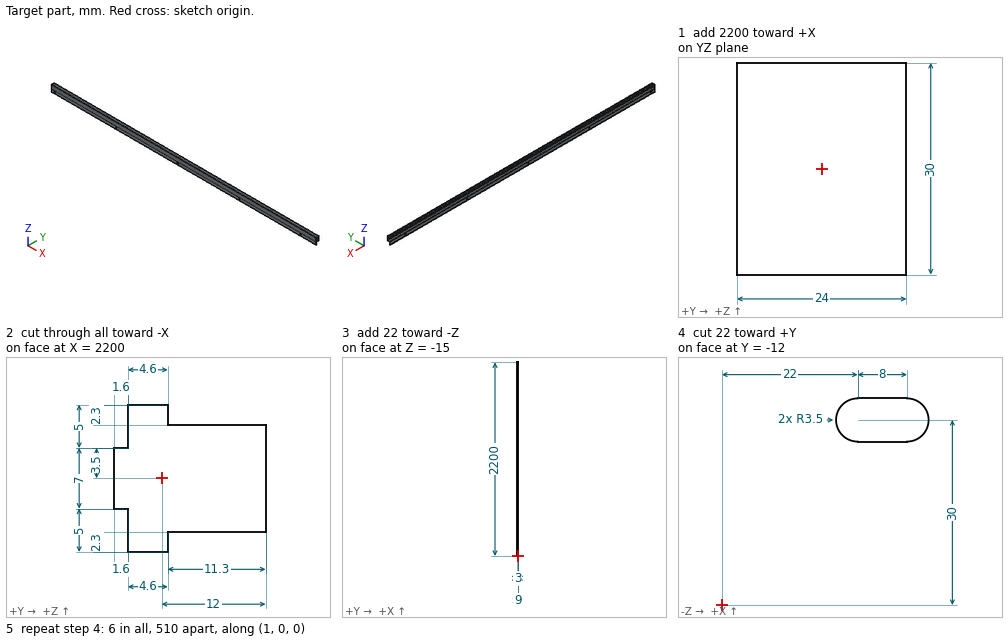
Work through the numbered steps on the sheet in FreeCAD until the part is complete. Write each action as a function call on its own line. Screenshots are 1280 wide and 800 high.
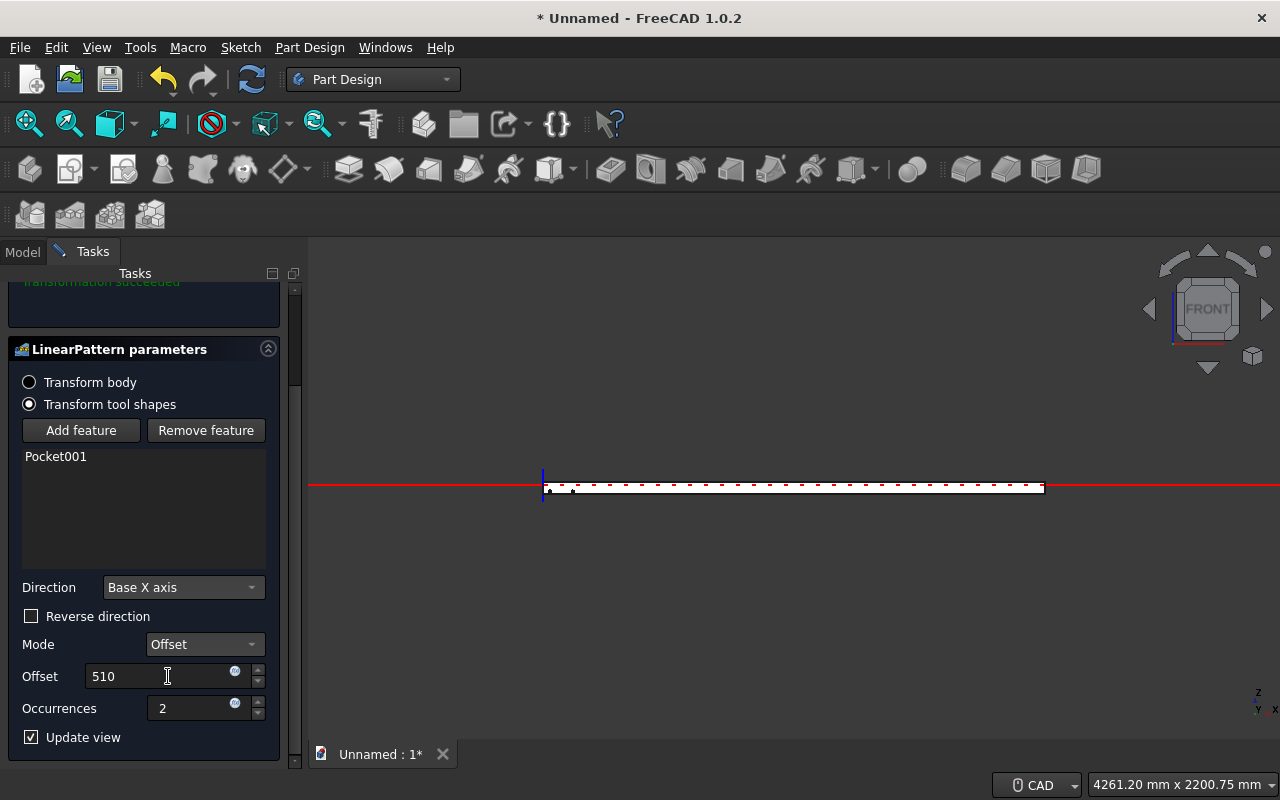
triple_click(198, 708)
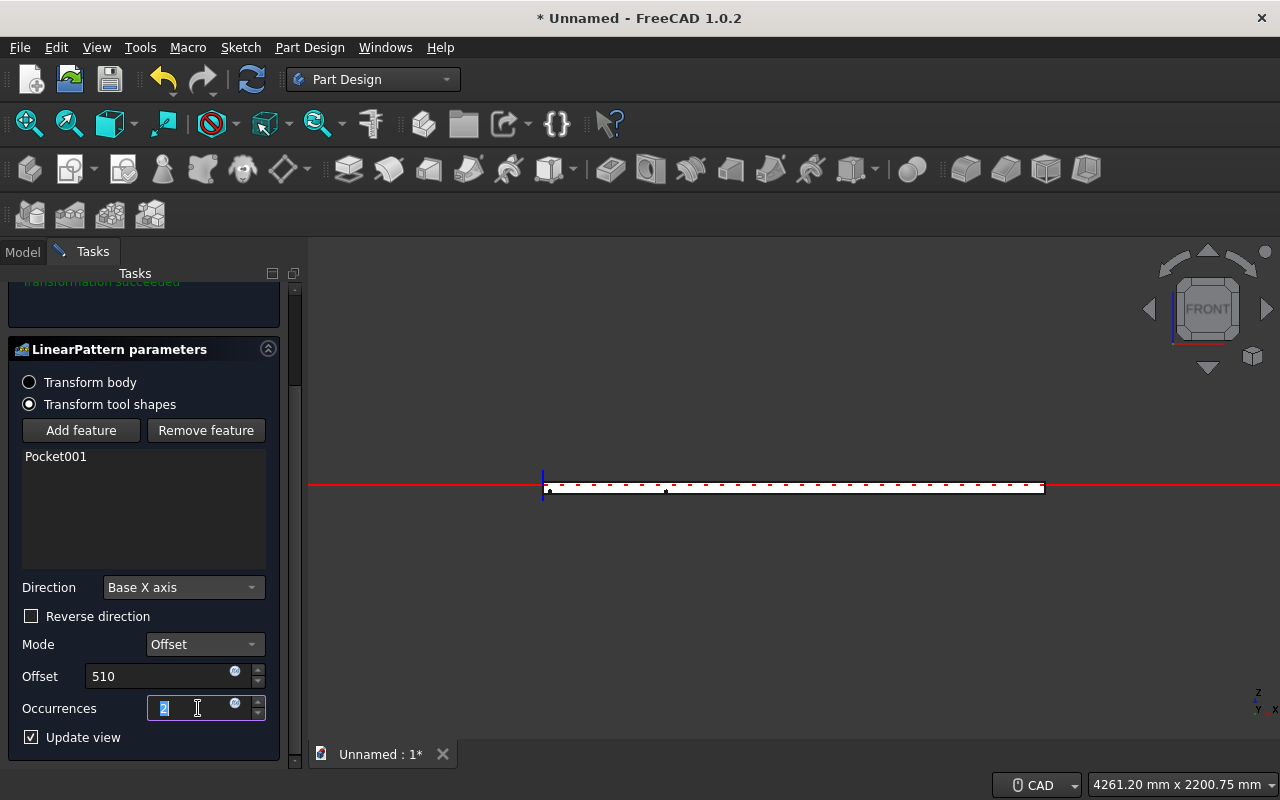
text(6)
key(Tab)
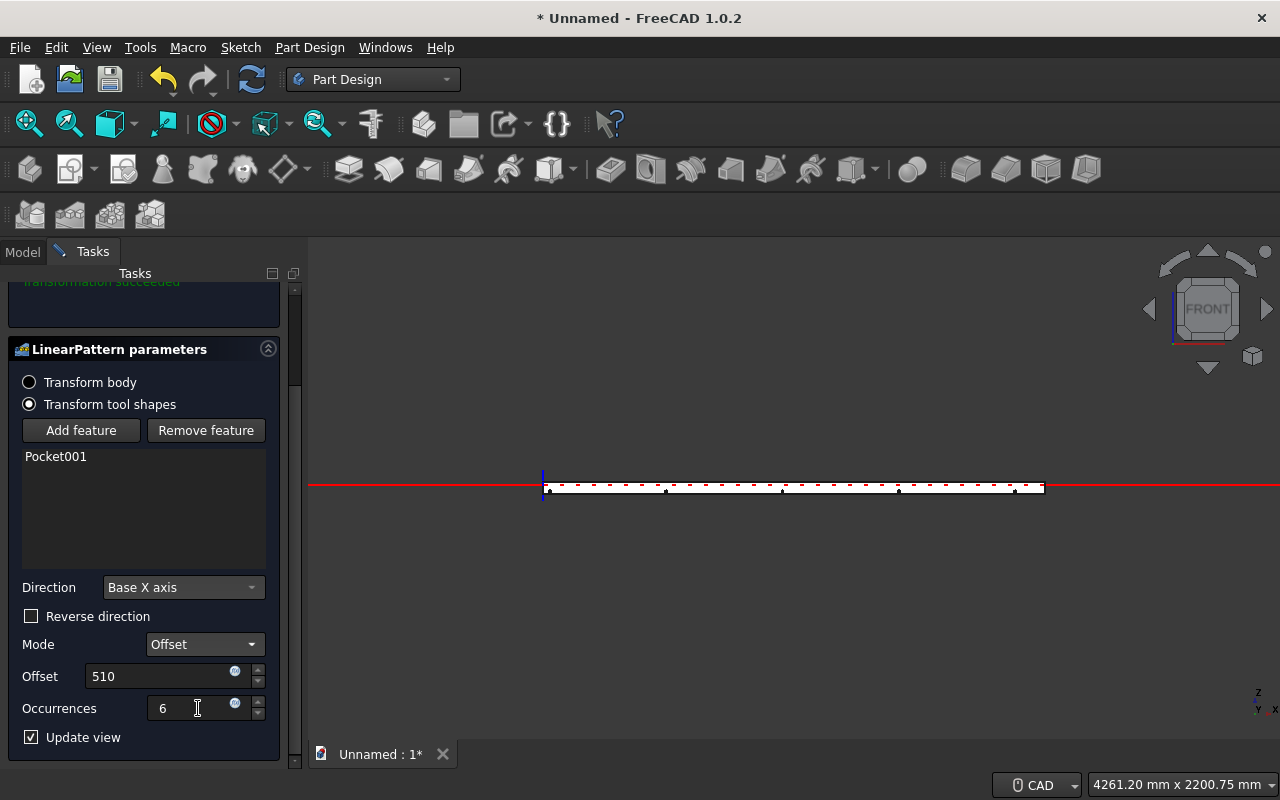
scroll(295, 526, up, 3)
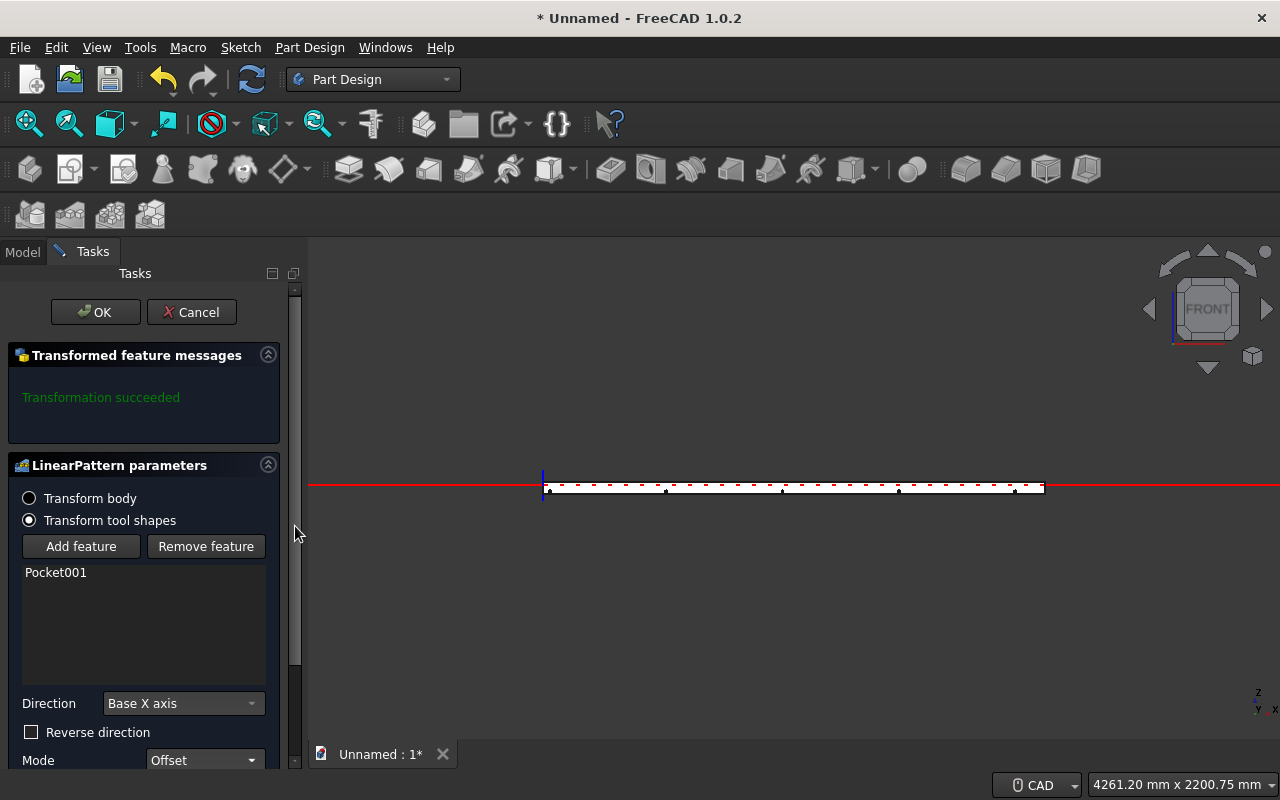
click(96, 312)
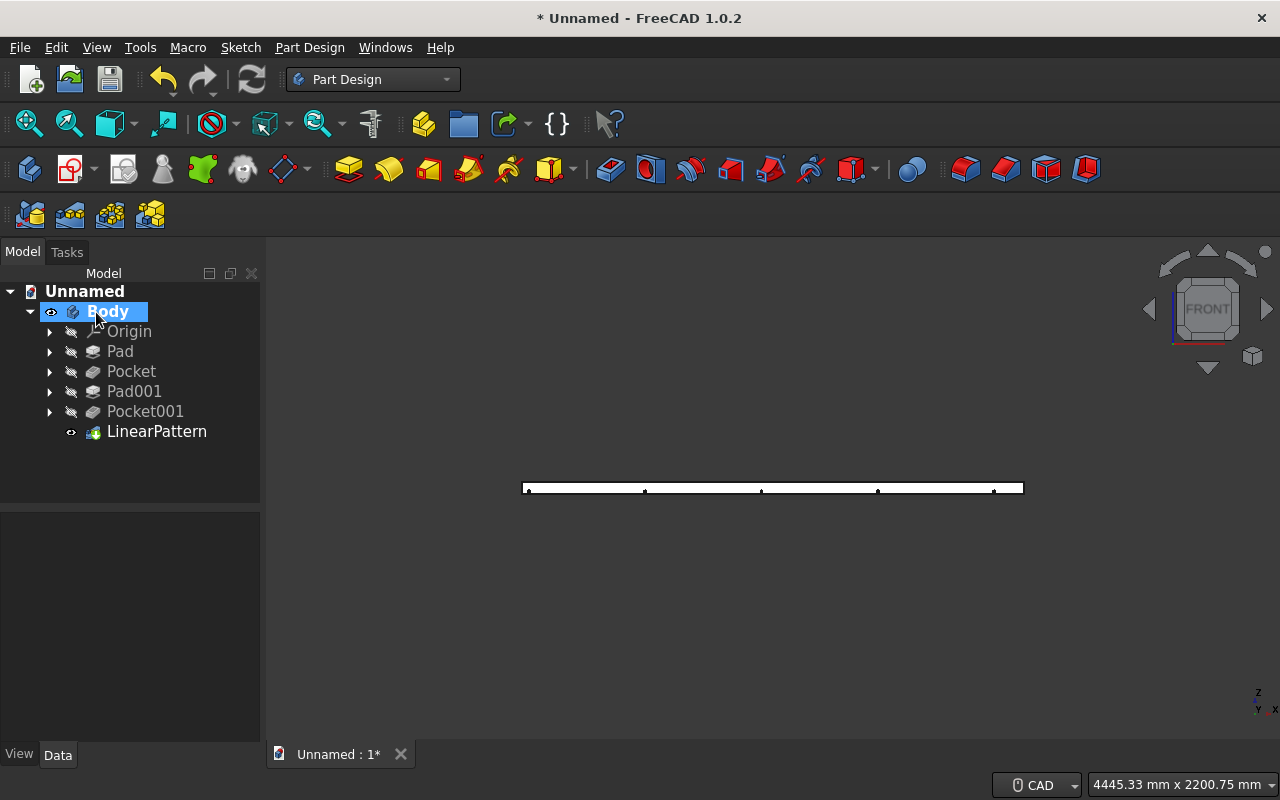
key(0)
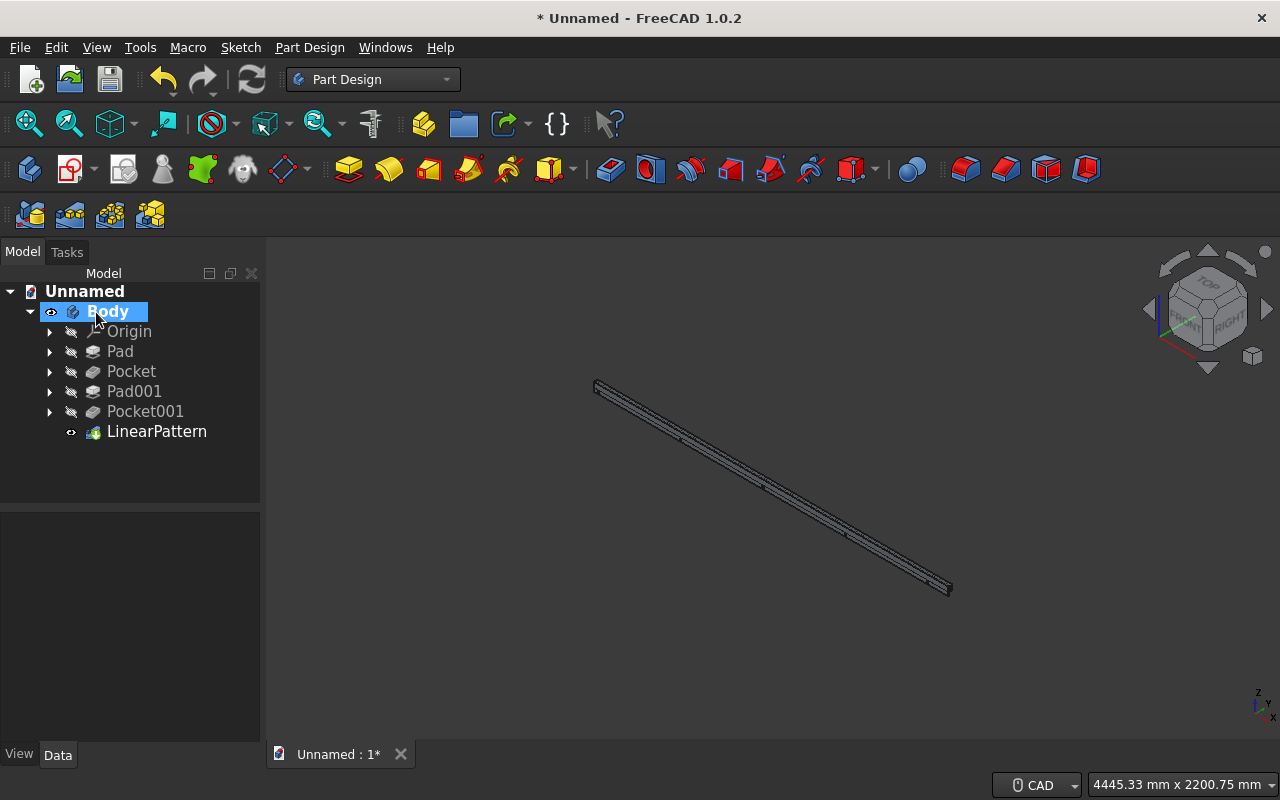
click(30, 124)